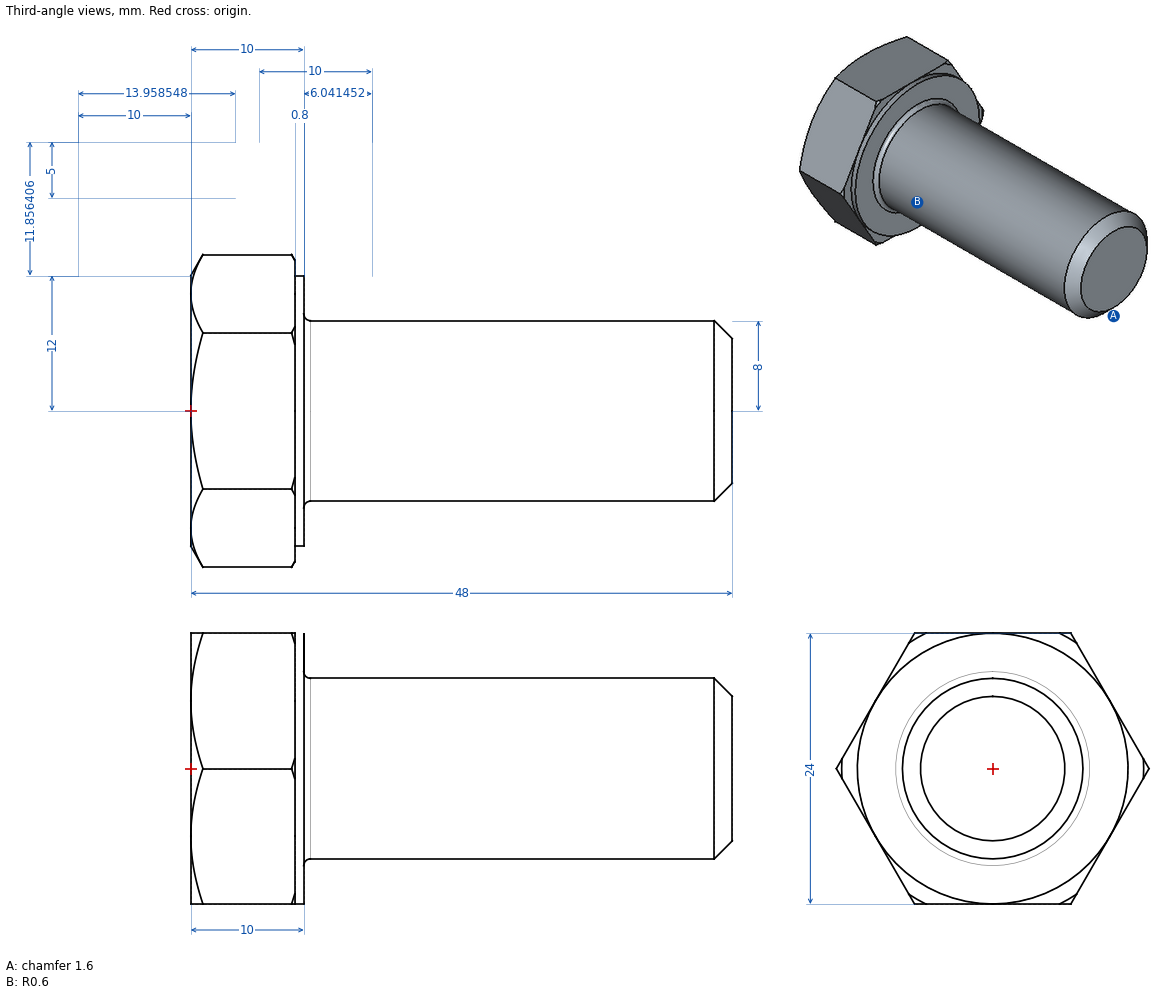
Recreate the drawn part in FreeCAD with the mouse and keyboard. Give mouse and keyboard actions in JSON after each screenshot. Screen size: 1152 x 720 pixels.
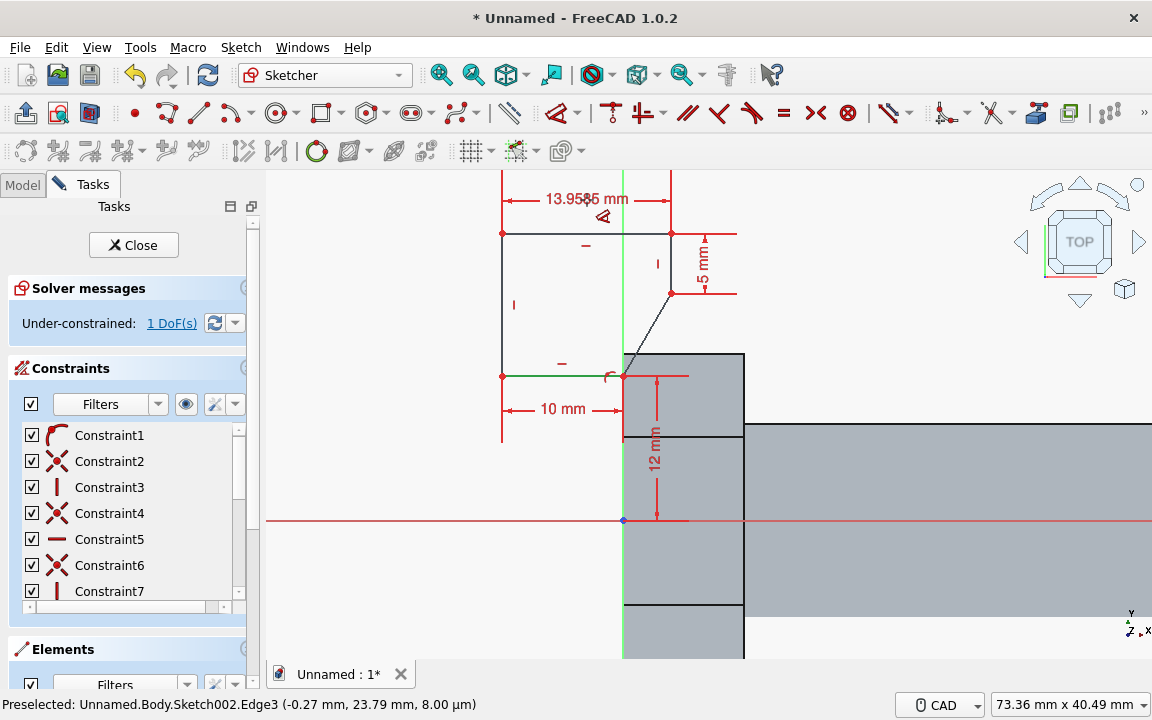
{"action": "left_click", "coordinate": [502, 276]}
{"action": "left_click", "coordinate": [468, 305]}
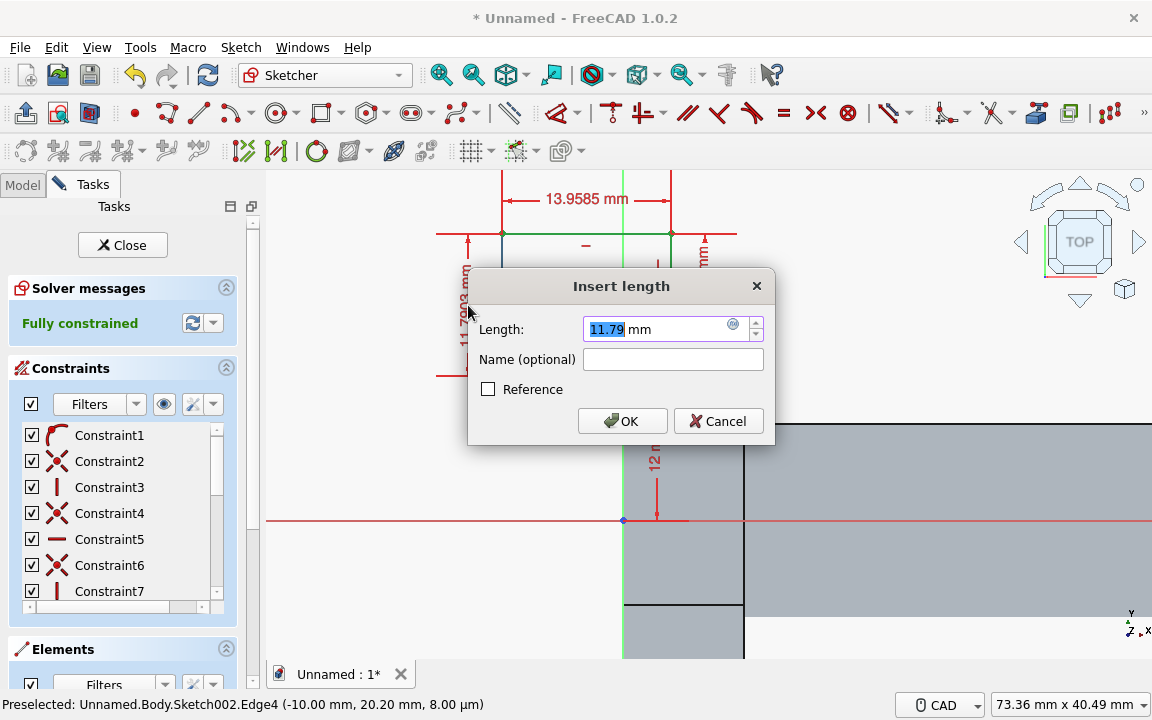
{"action": "type", "text": "11.856406"}
{"action": "key", "text": "Return"}
{"action": "key", "text": "Escape"}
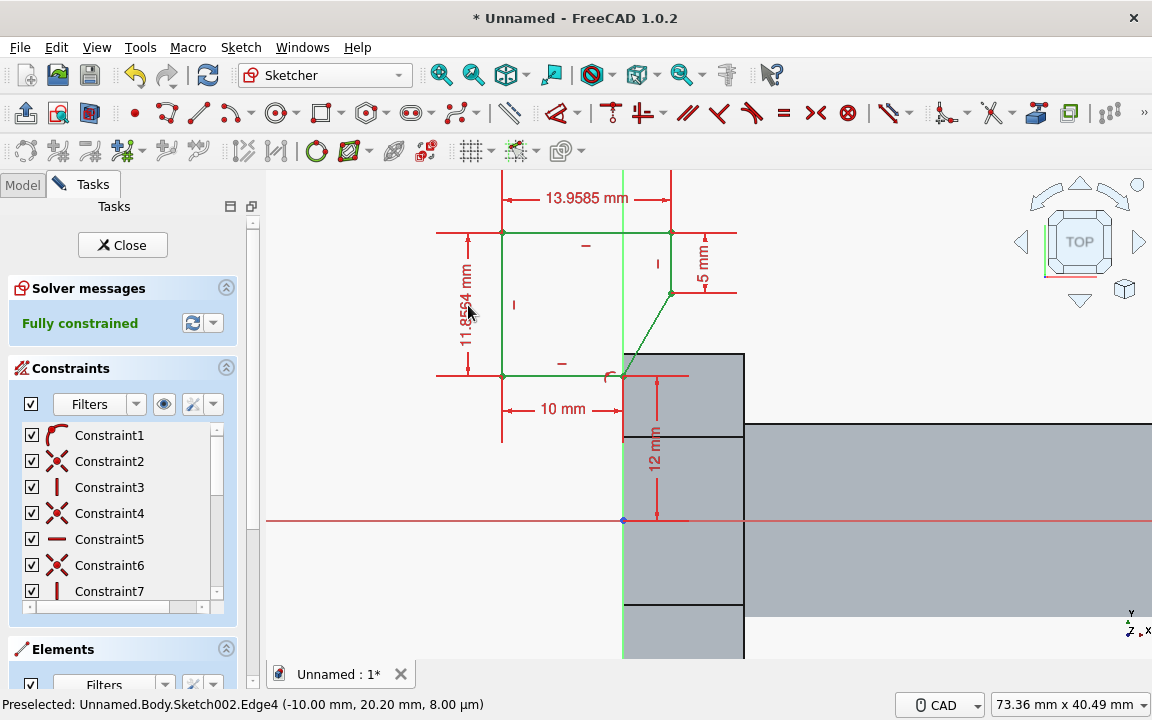
{"action": "left_click", "coordinate": [123, 245]}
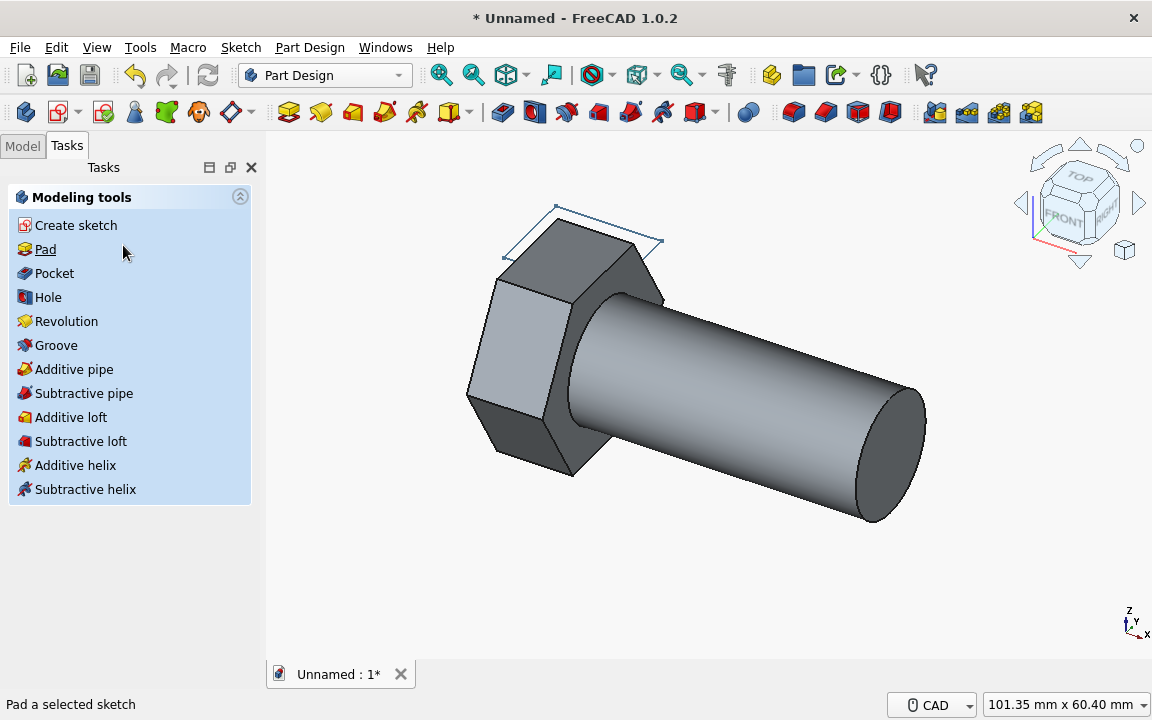
{"action": "left_click", "coordinate": [568, 112]}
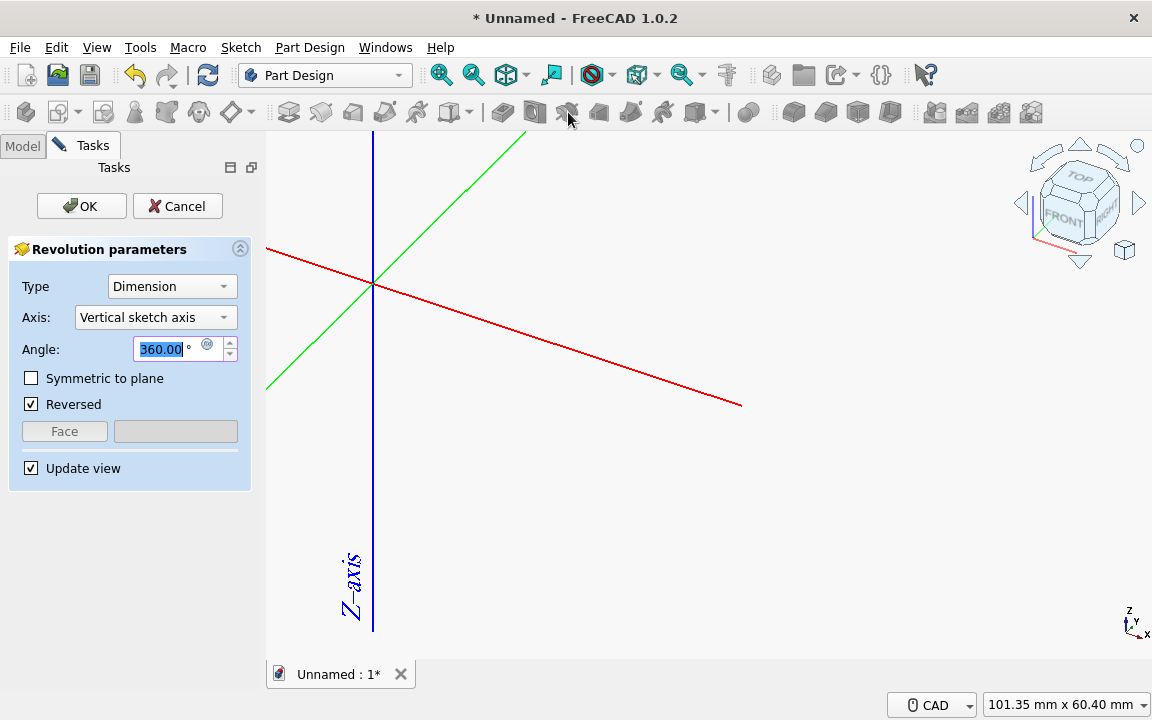
{"action": "left_click", "coordinate": [156, 318]}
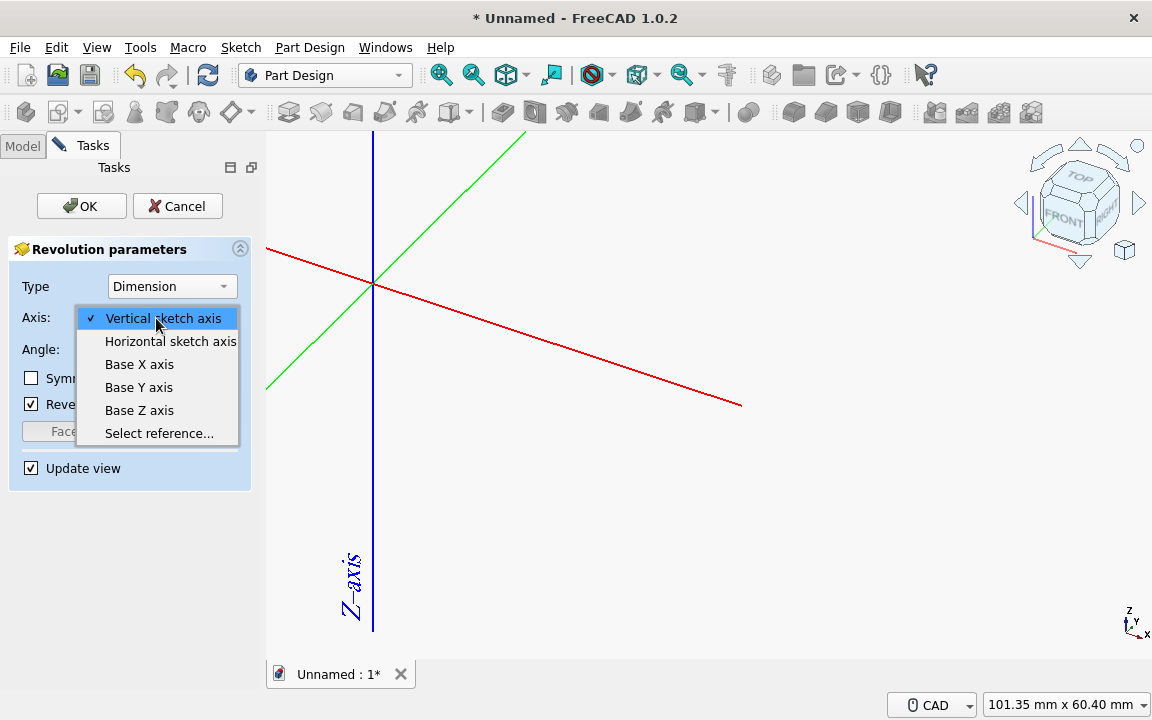
{"action": "left_click", "coordinate": [156, 342]}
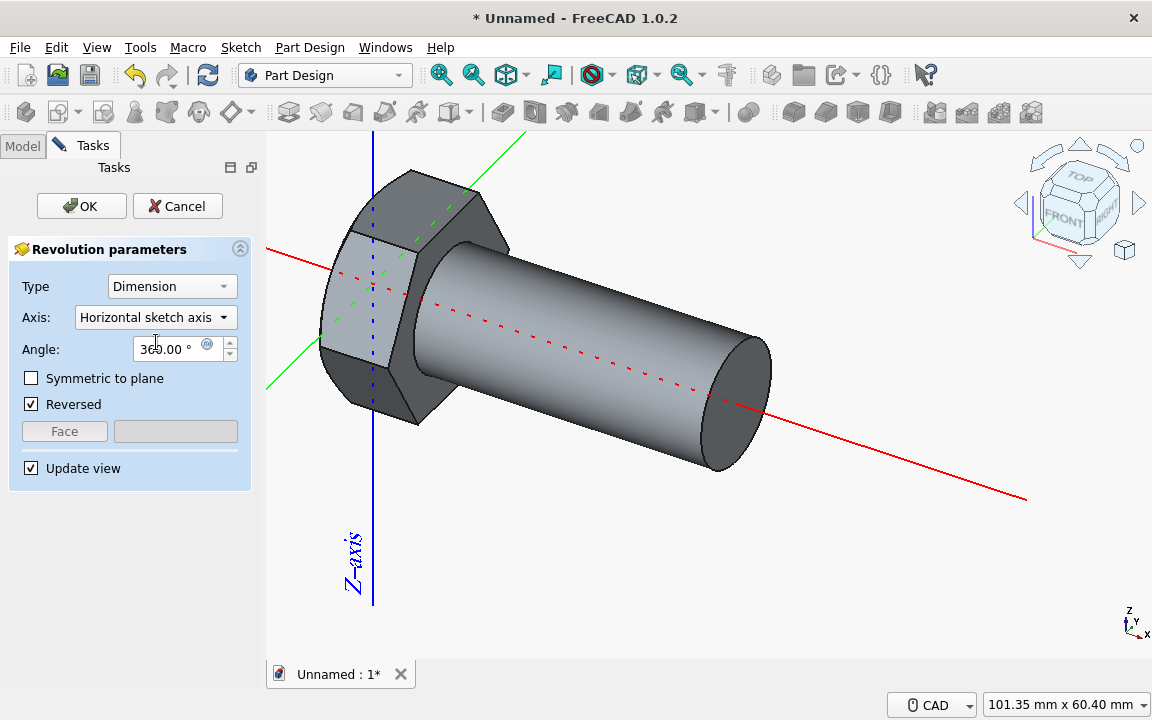
{"action": "left_click", "coordinate": [82, 206]}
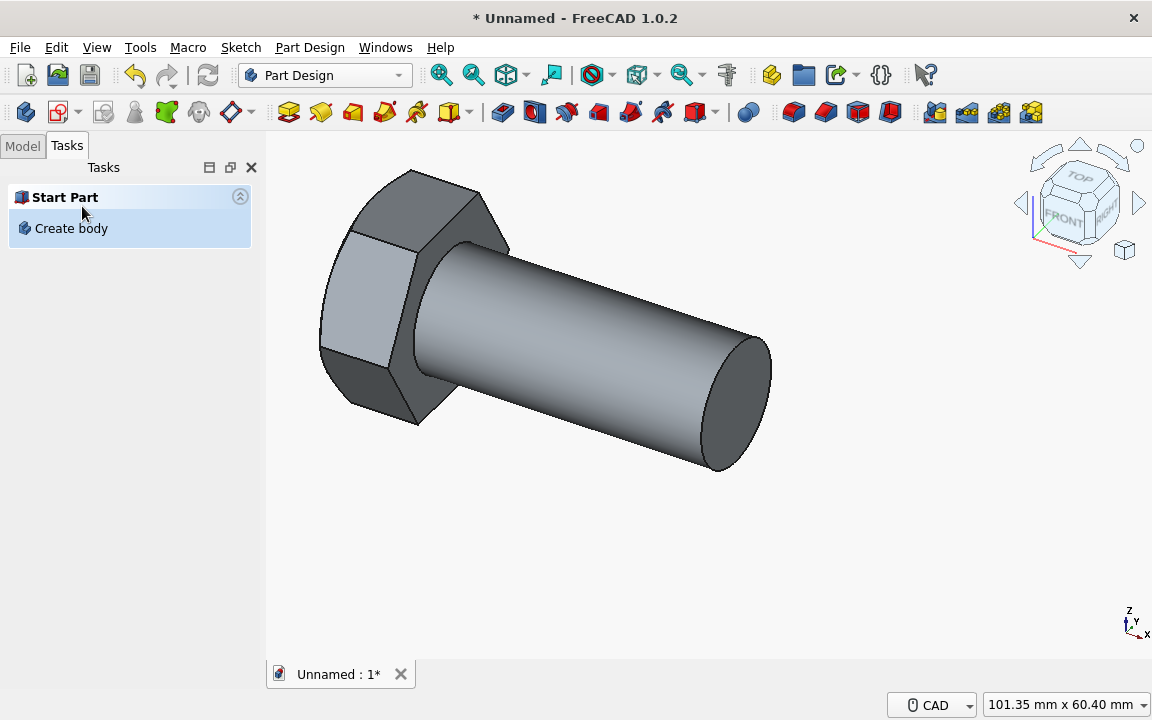
{"action": "left_click", "coordinate": [58, 112]}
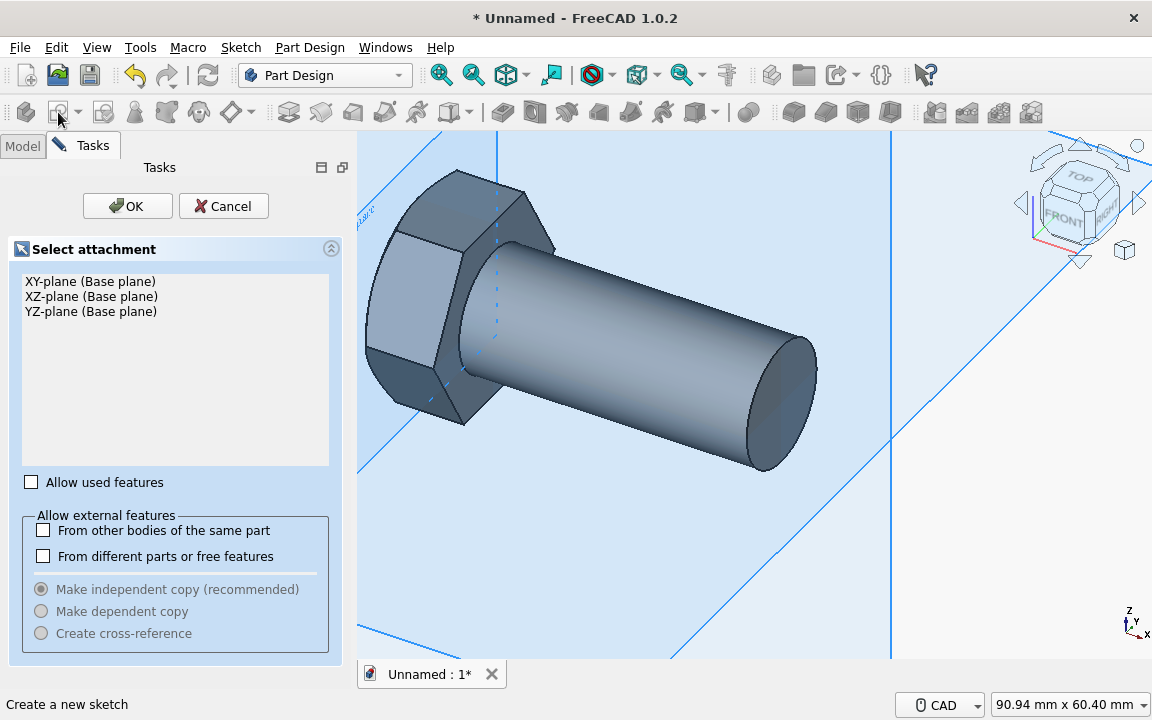
{"action": "left_click", "coordinate": [82, 282]}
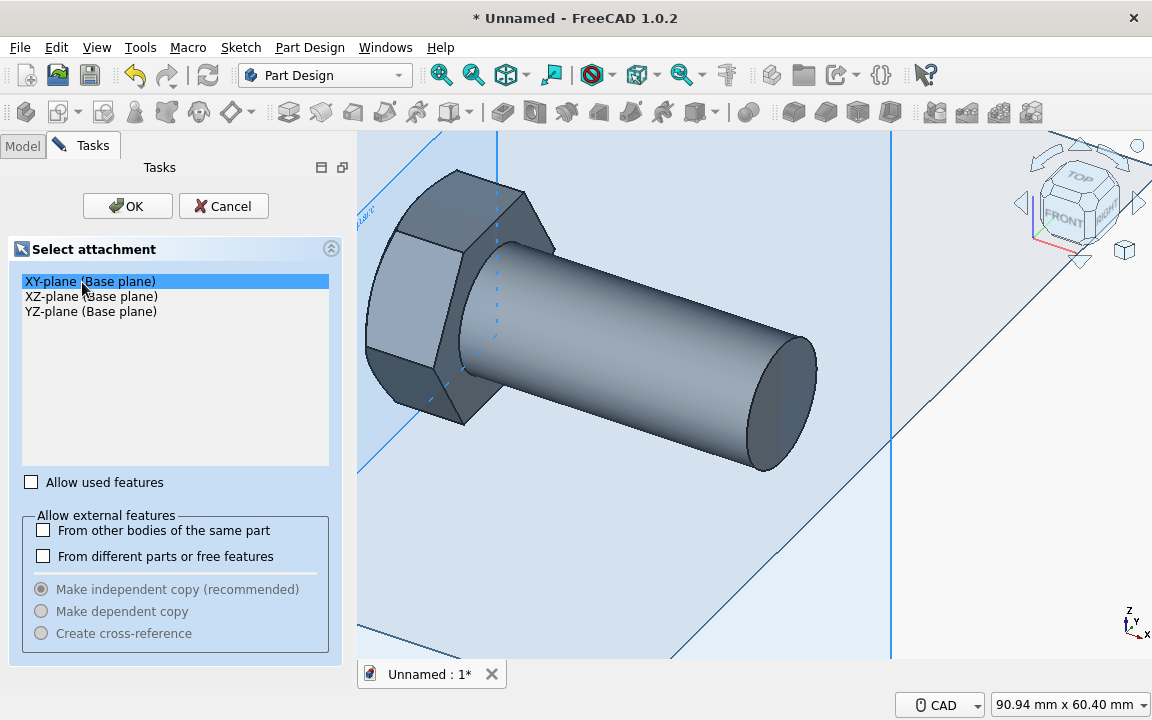
{"action": "left_click", "coordinate": [128, 206]}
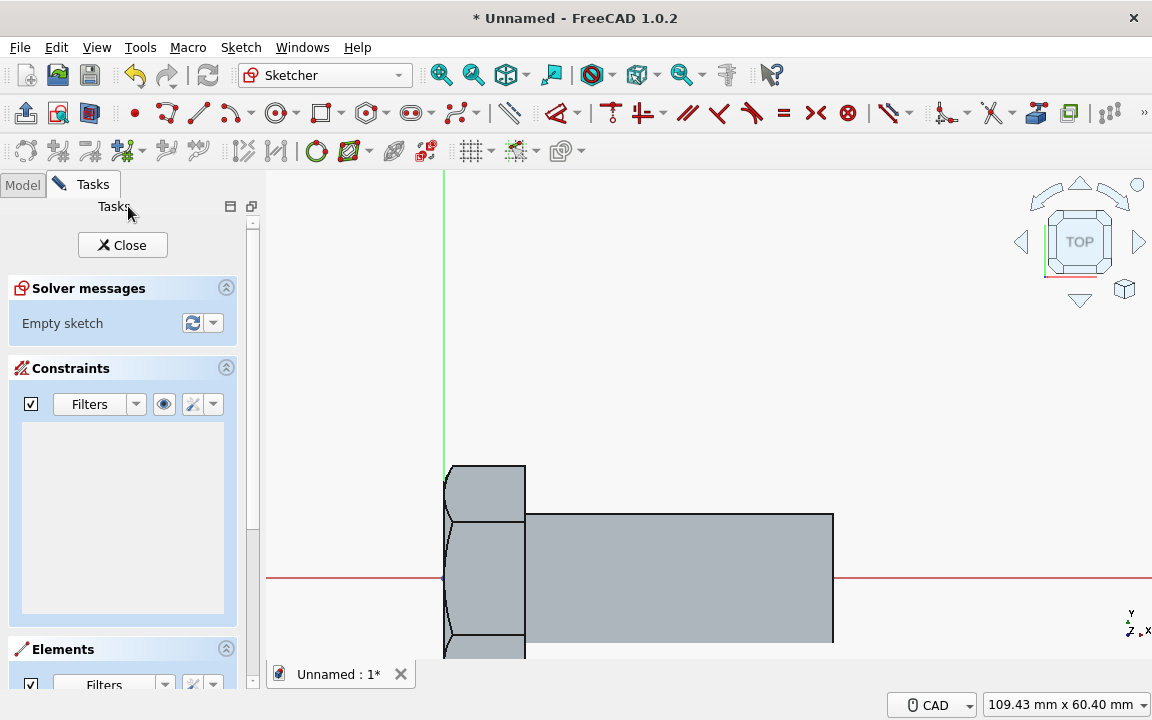
{"action": "left_click", "coordinate": [90, 114]}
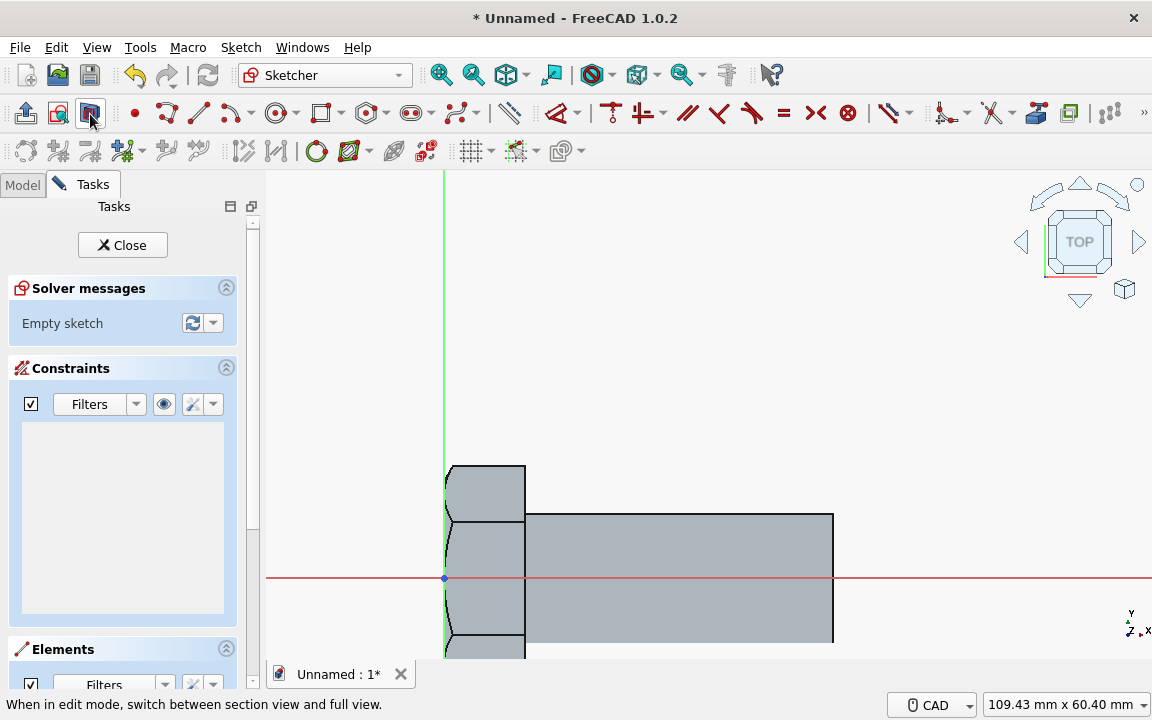
{"action": "scroll", "coordinate": [294, 619], "scroll_direction": "up", "scroll_amount": 2}